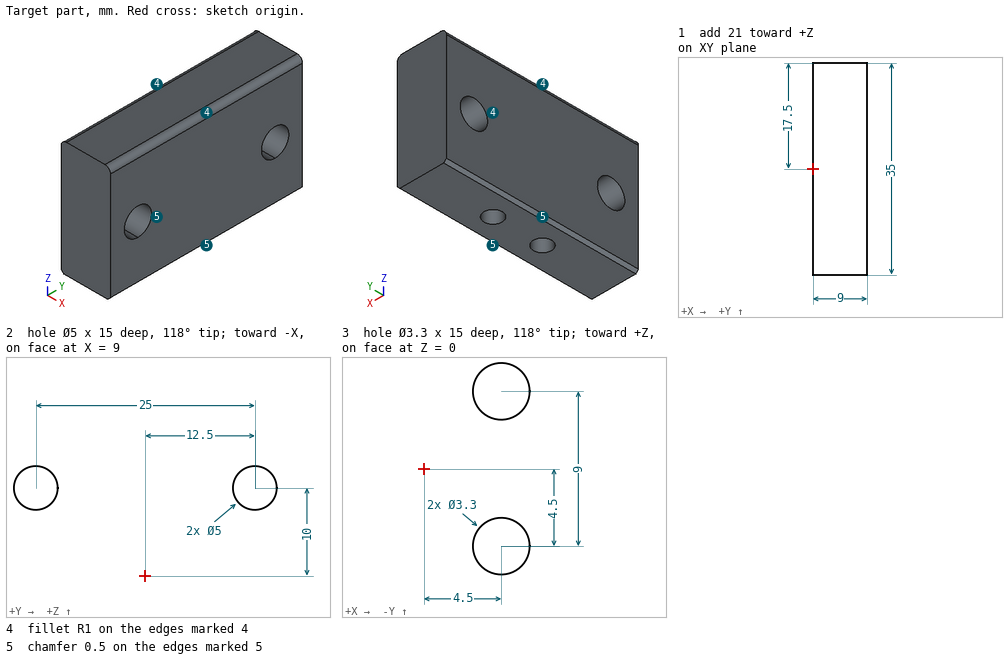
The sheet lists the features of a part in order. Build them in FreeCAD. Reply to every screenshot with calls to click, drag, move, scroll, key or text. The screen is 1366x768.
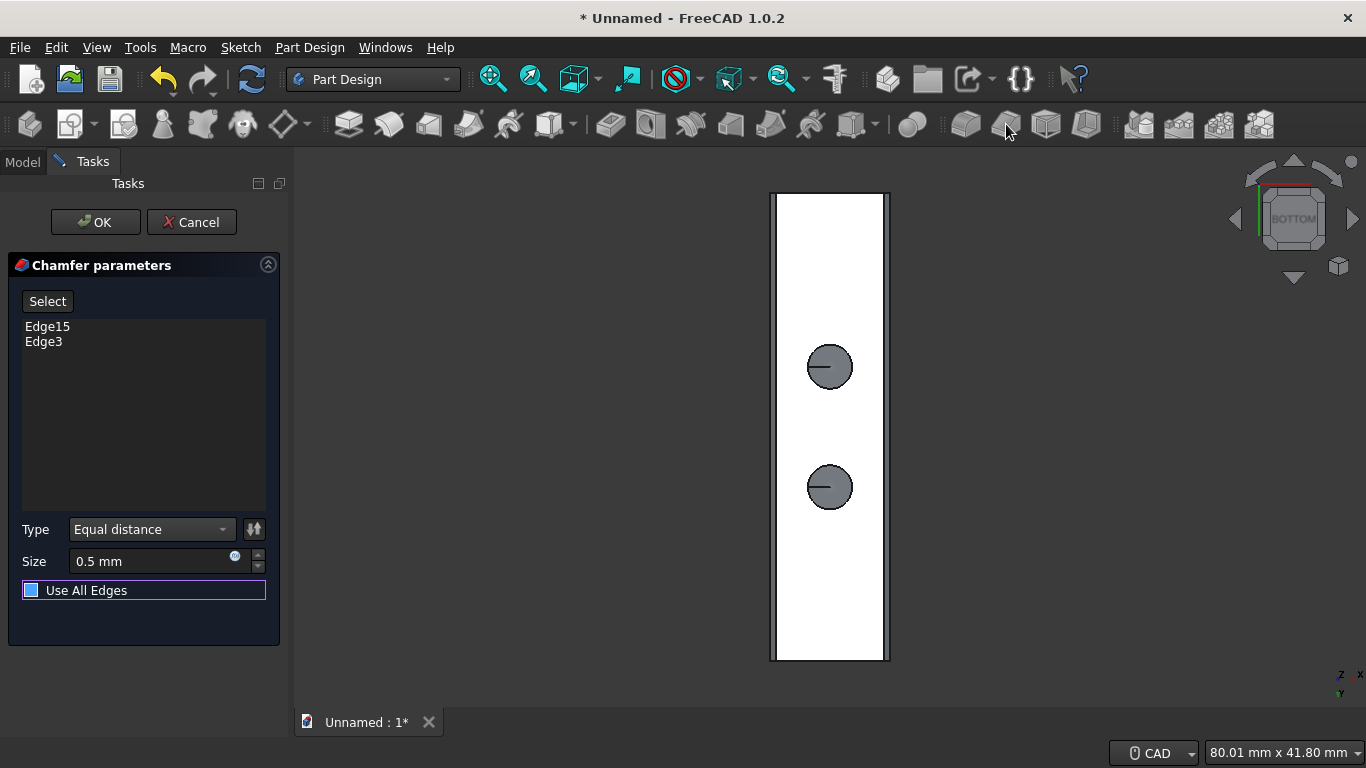
click(96, 222)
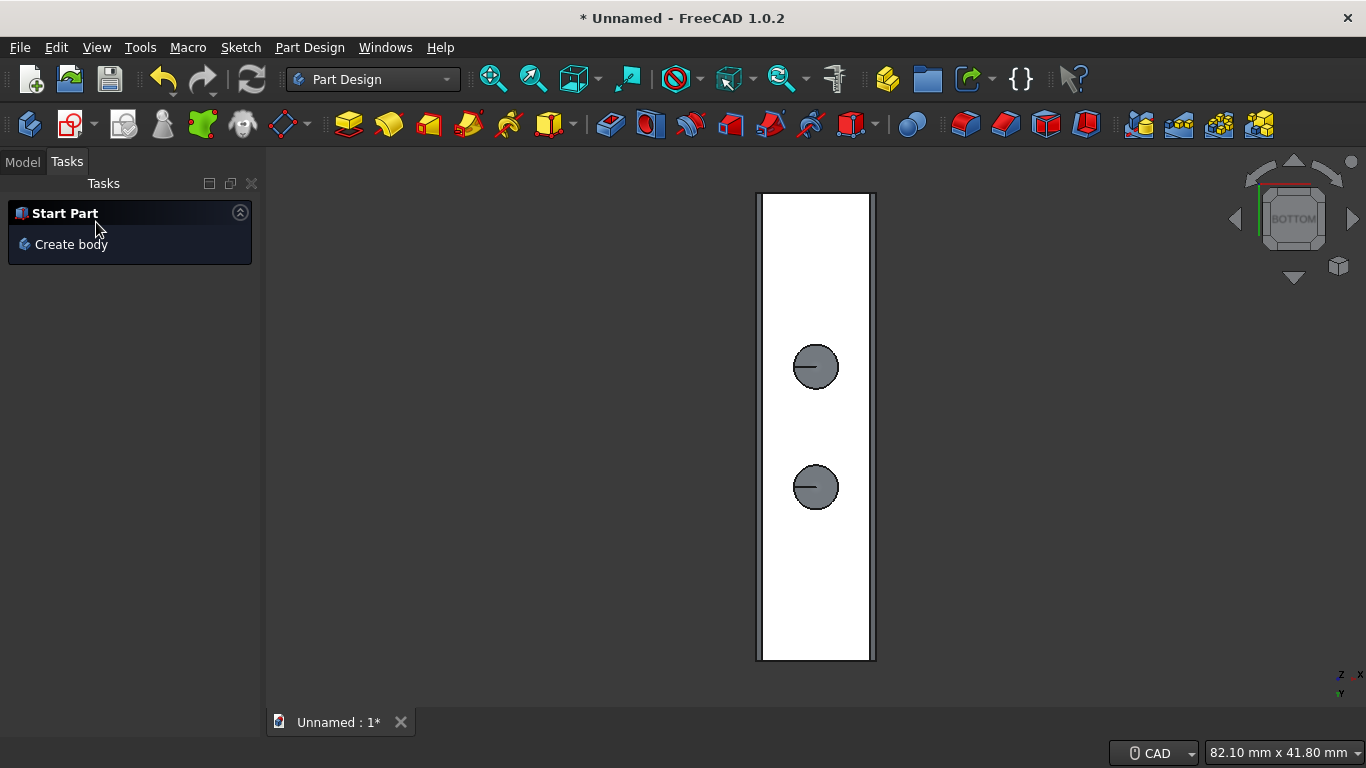
key(0)